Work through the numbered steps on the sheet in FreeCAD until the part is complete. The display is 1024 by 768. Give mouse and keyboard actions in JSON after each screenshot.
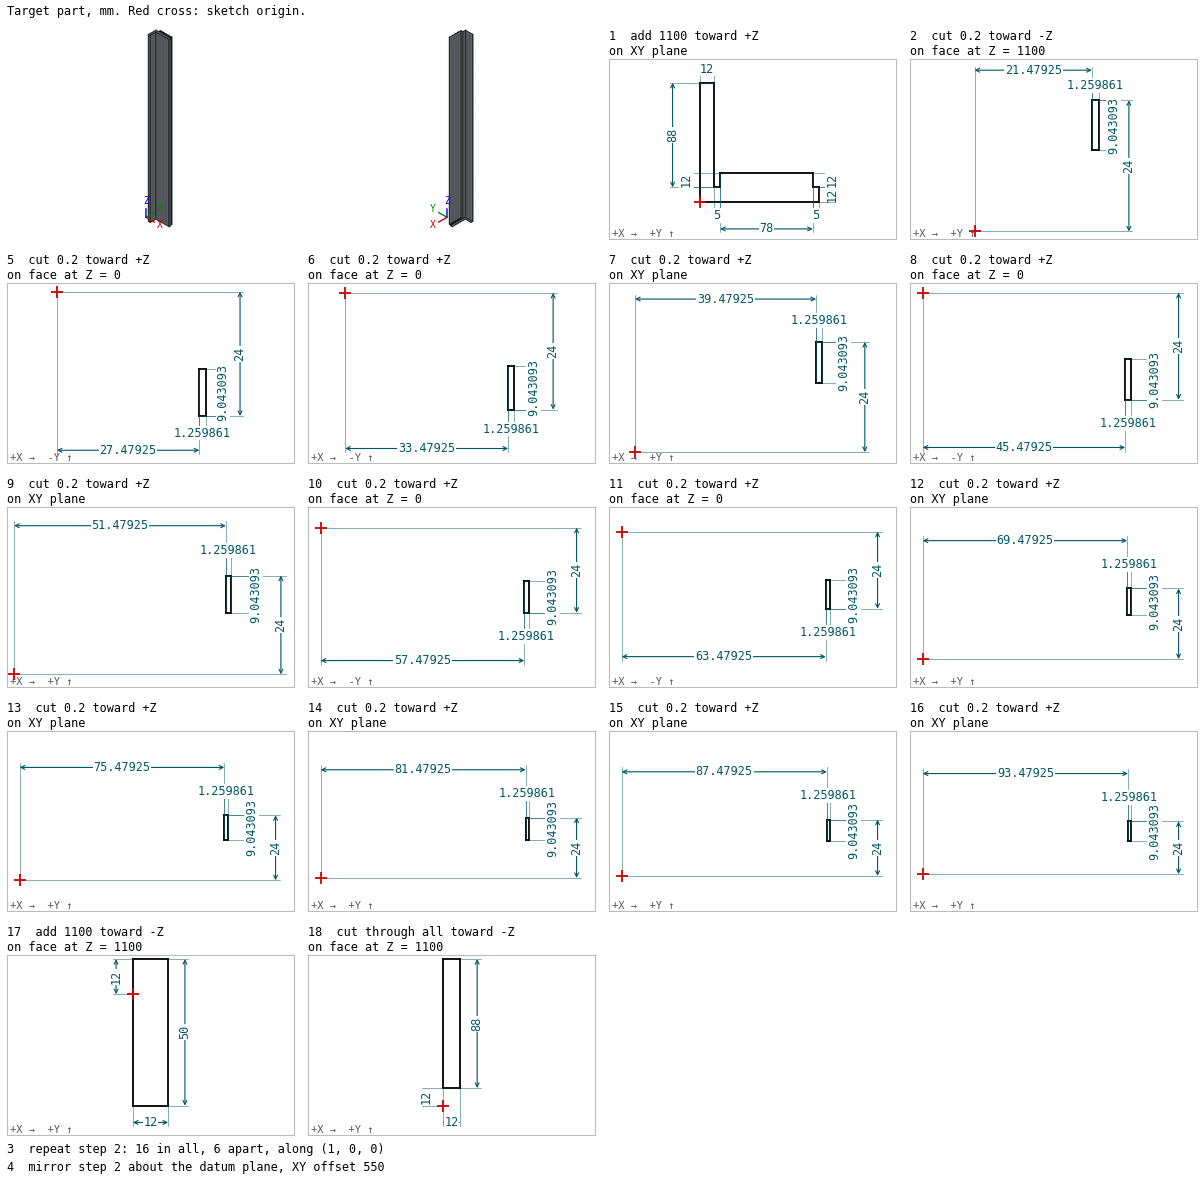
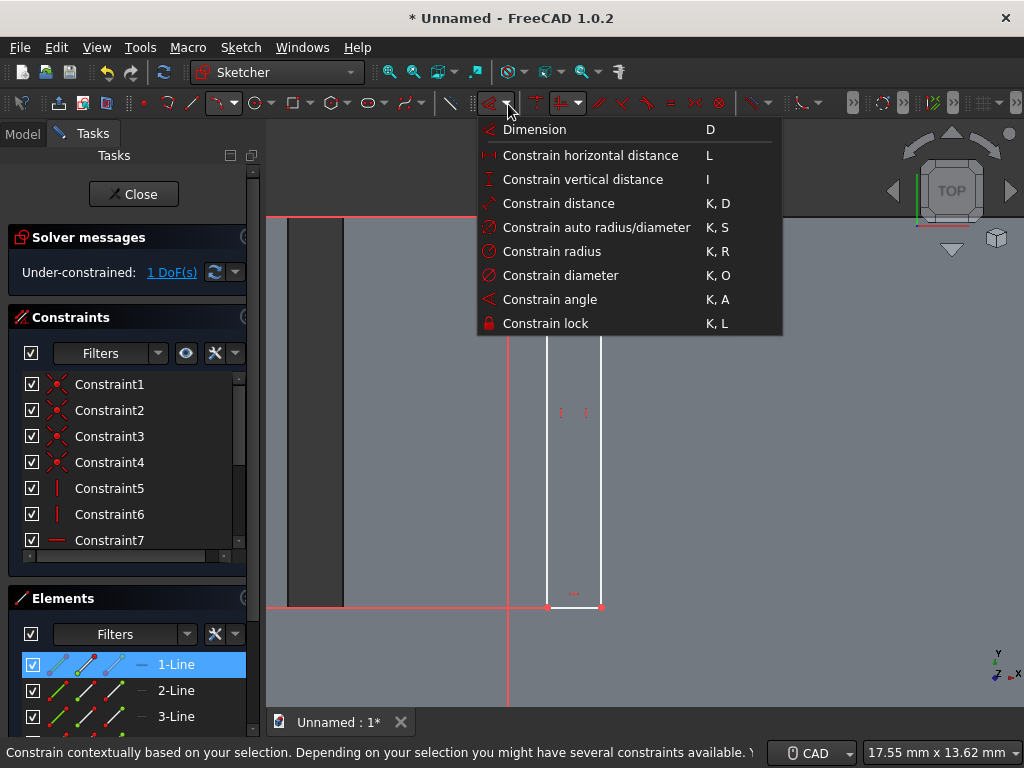
{"action": "left_click", "coordinate": [630, 155]}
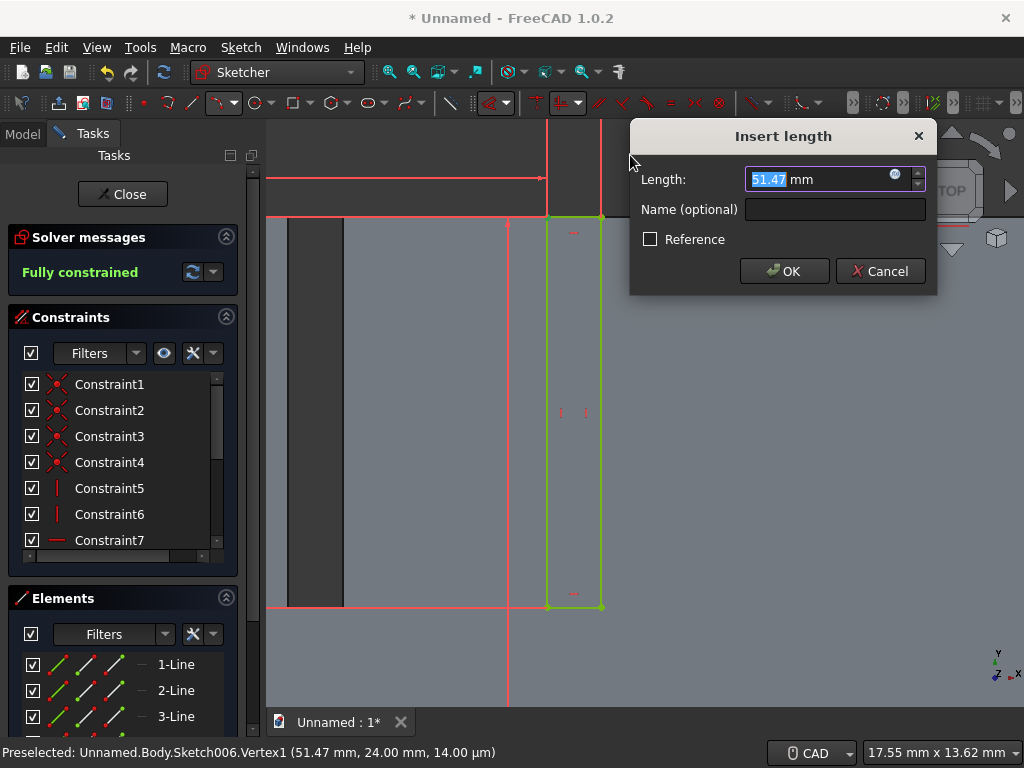
{"action": "type", "text": "51.47925"}
{"action": "key", "text": "Return"}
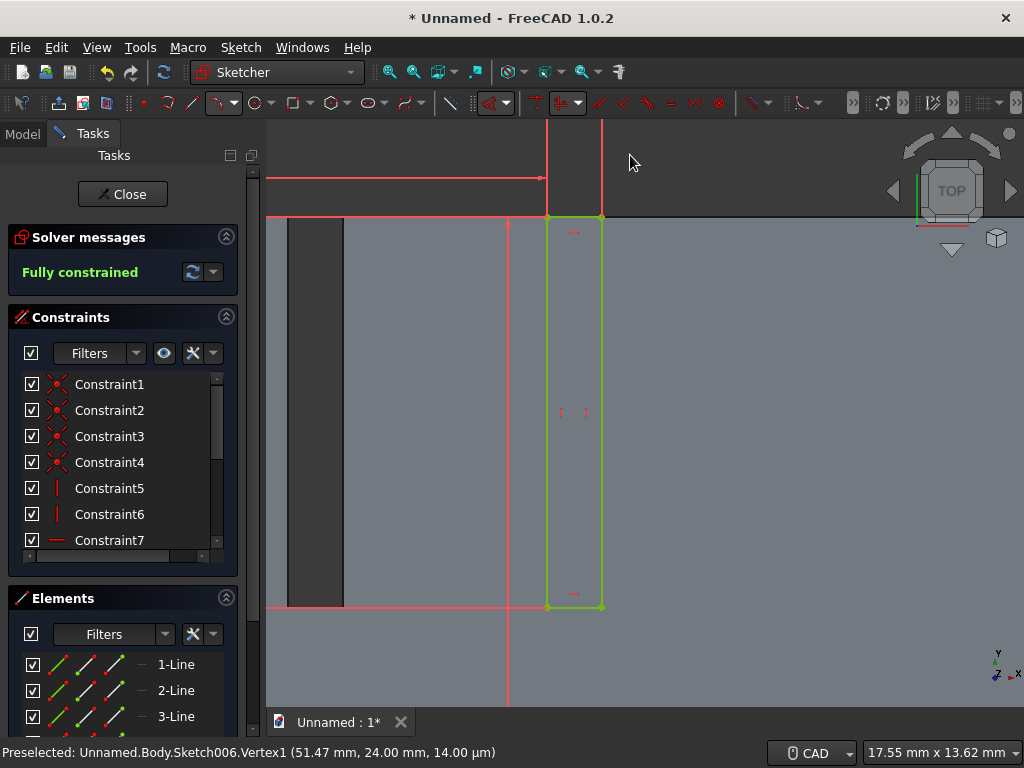
{"action": "left_click", "coordinate": [123, 194]}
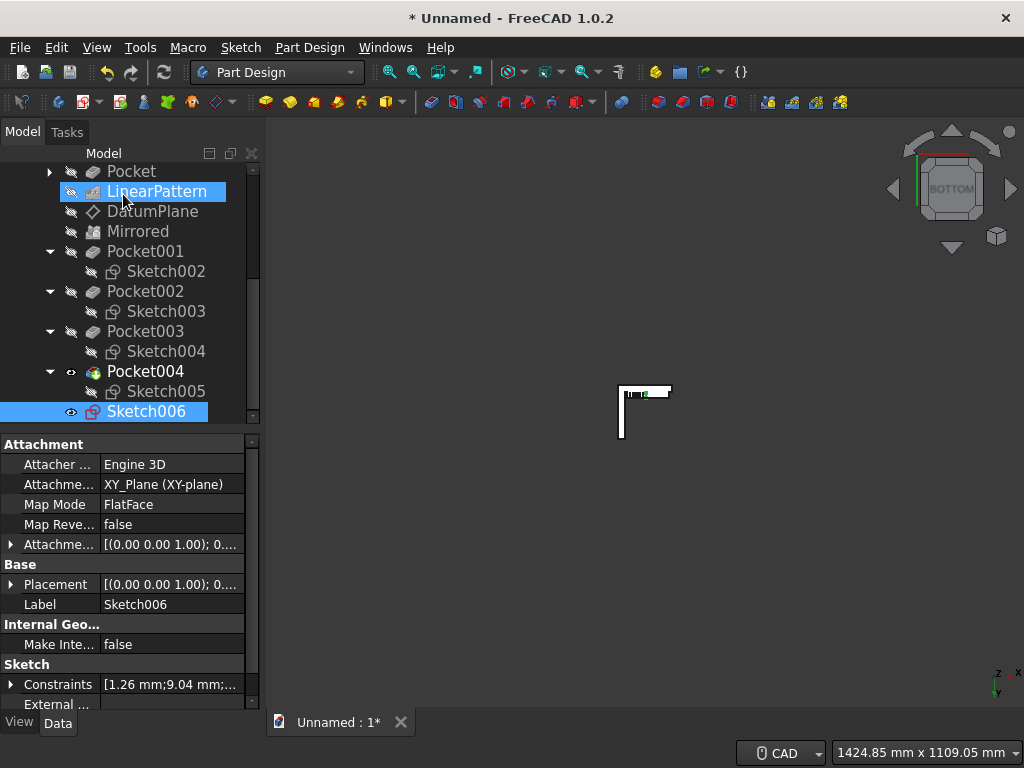
{"action": "left_click", "coordinate": [432, 102]}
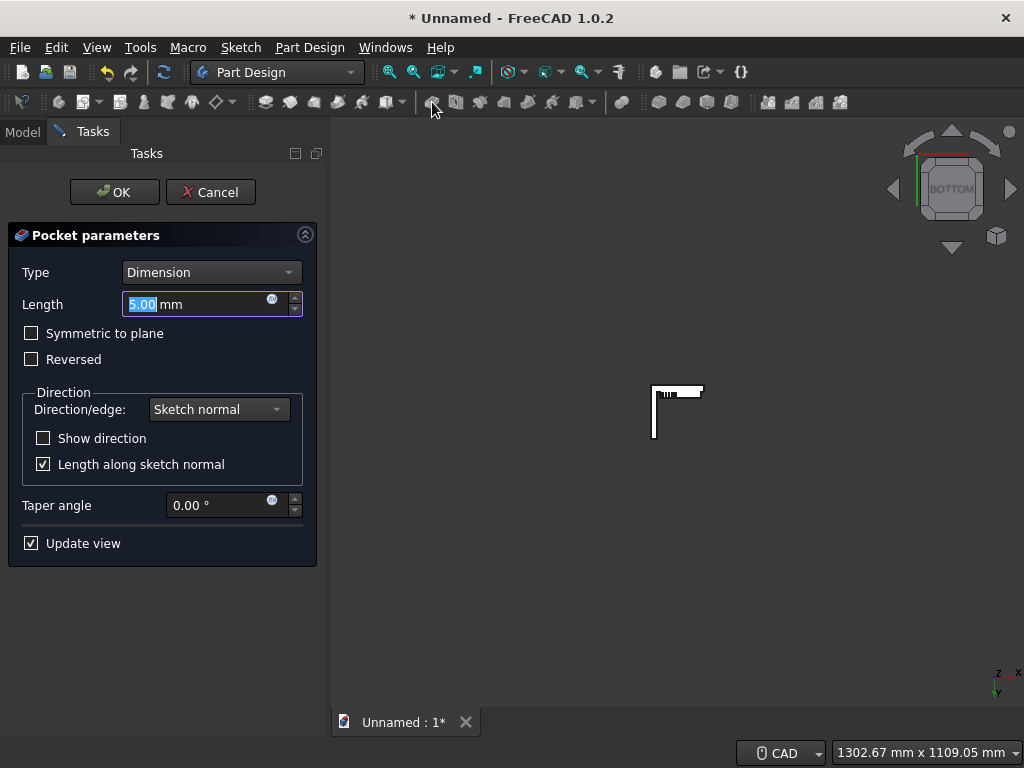
{"action": "type", "text": "0.2"}
{"action": "key", "text": "Tab"}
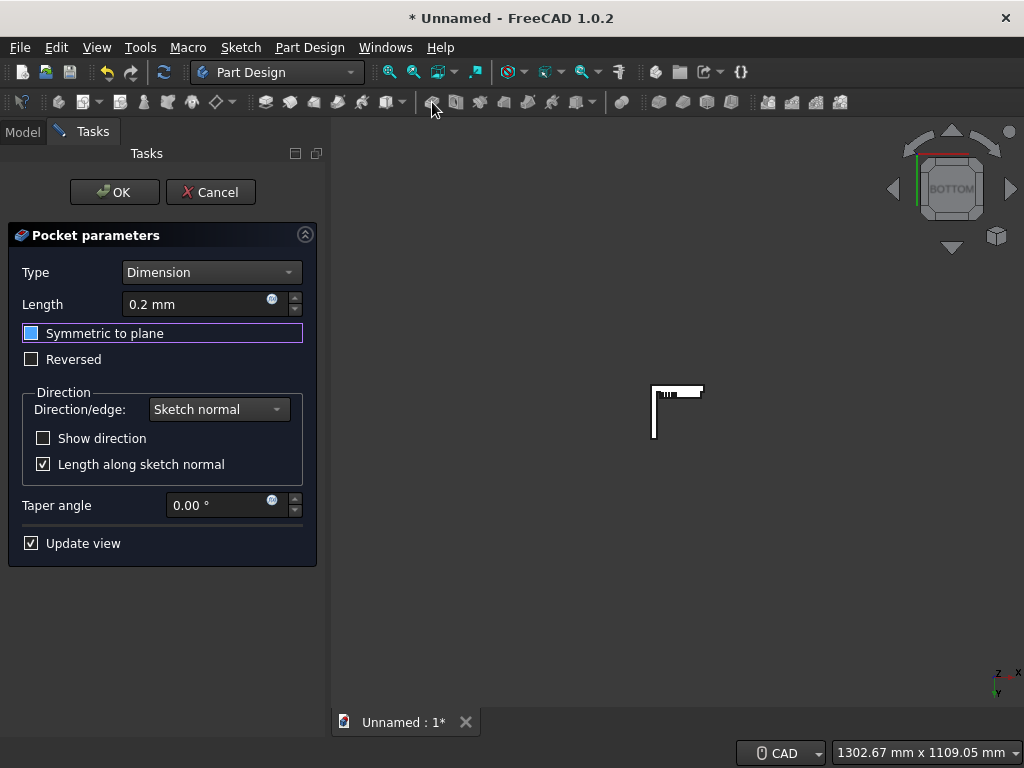
{"action": "left_click", "coordinate": [30, 359]}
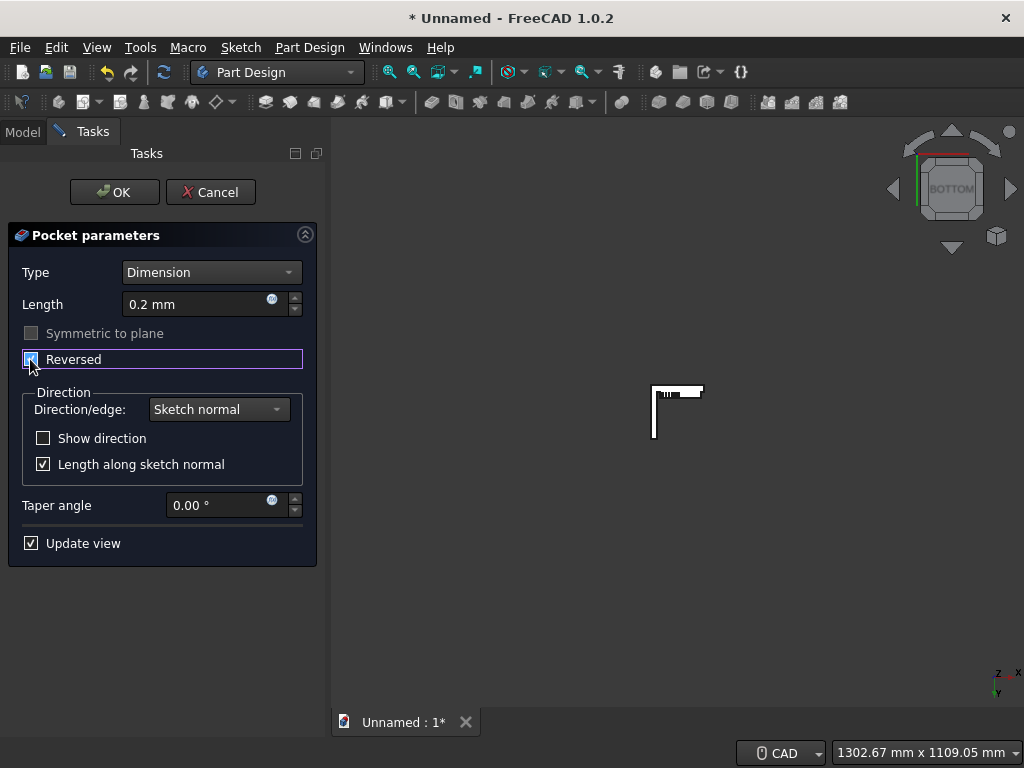
{"action": "left_click", "coordinate": [115, 192]}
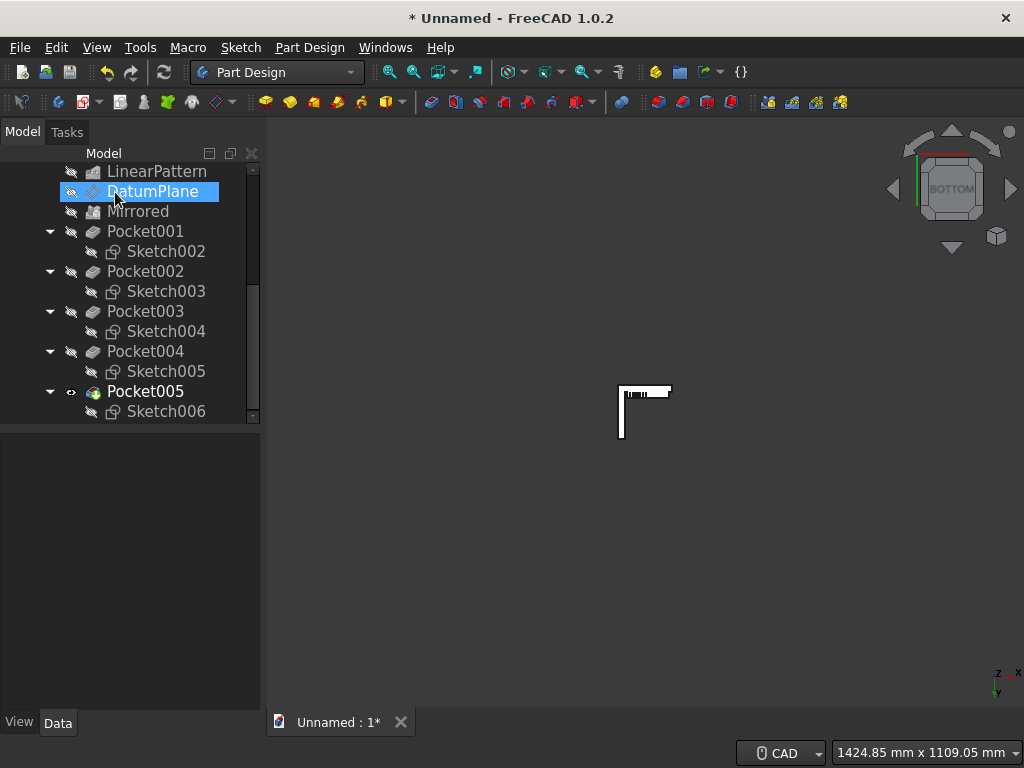
{"action": "left_click", "coordinate": [390, 72]}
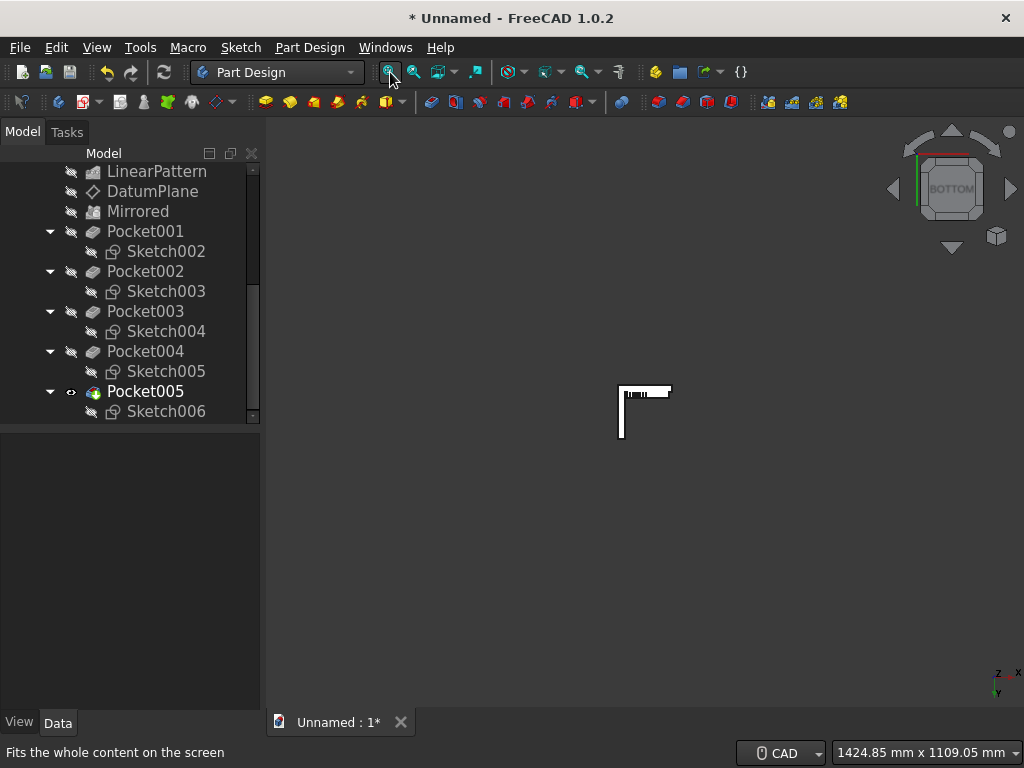
{"action": "left_click", "coordinate": [660, 388]}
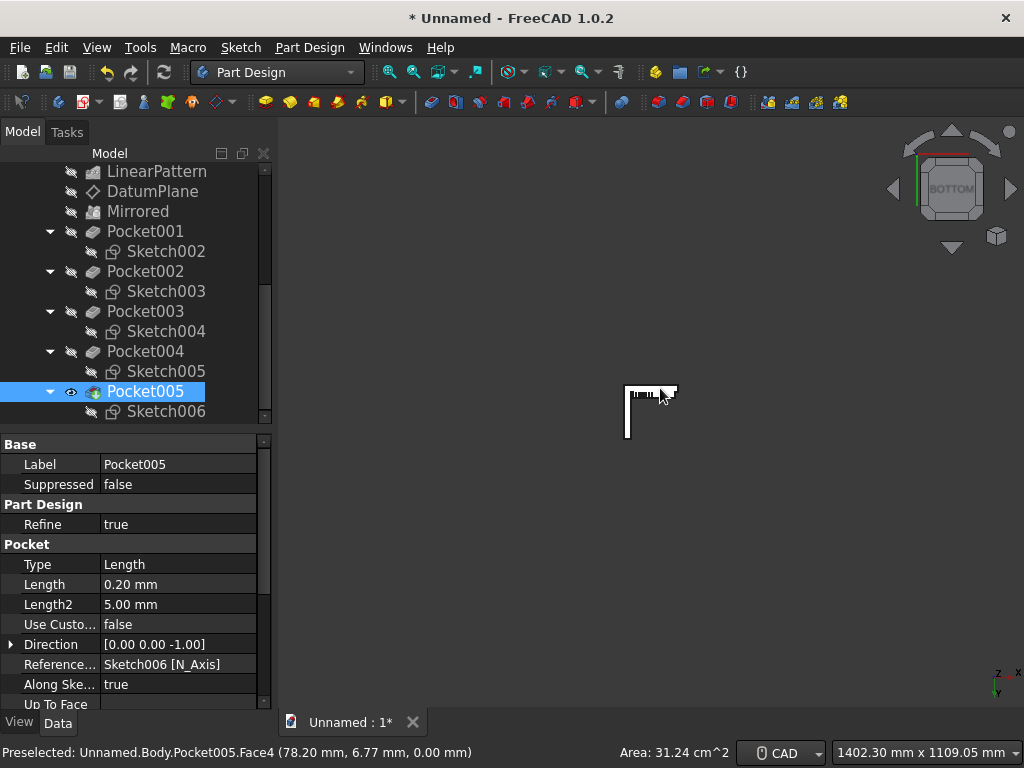
{"action": "left_click", "coordinate": [84, 102]}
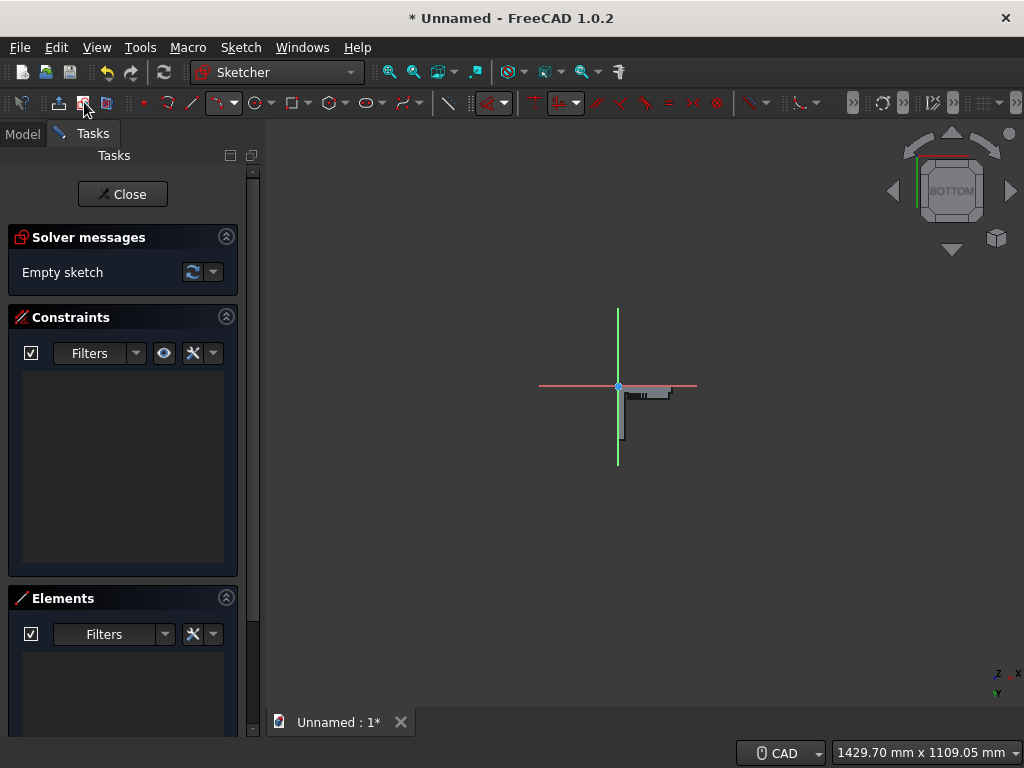
{"action": "scroll", "coordinate": [653, 396], "scroll_direction": "up", "scroll_amount": 15}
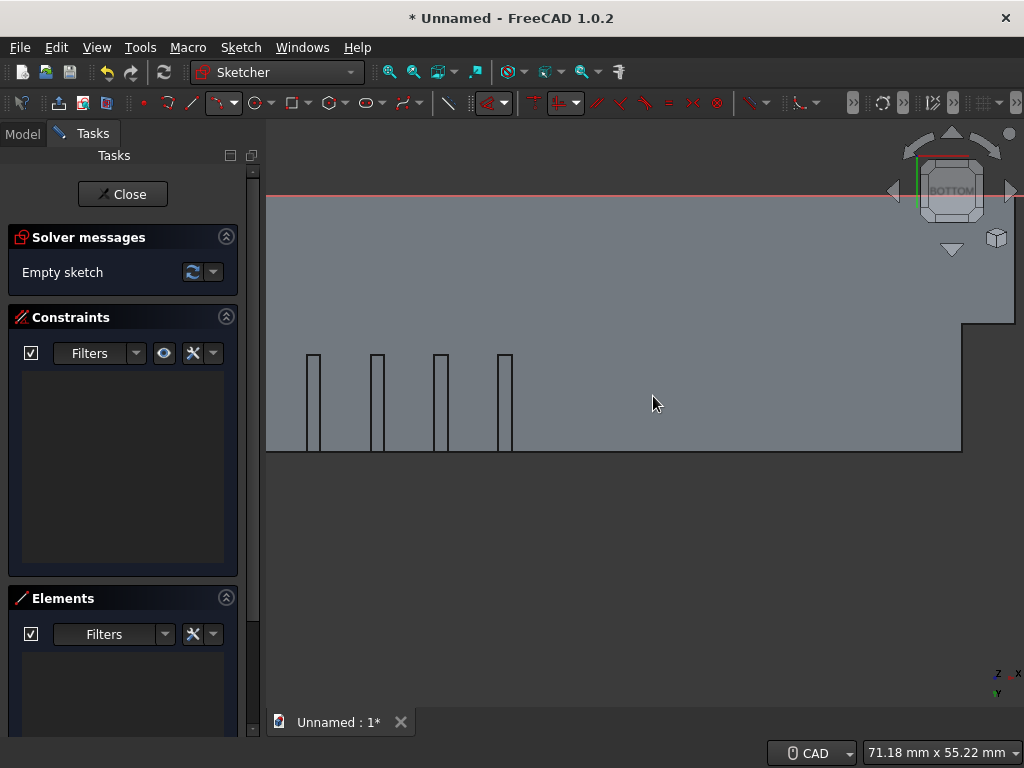
{"action": "scroll", "coordinate": [566, 400], "scroll_direction": "up", "scroll_amount": 7}